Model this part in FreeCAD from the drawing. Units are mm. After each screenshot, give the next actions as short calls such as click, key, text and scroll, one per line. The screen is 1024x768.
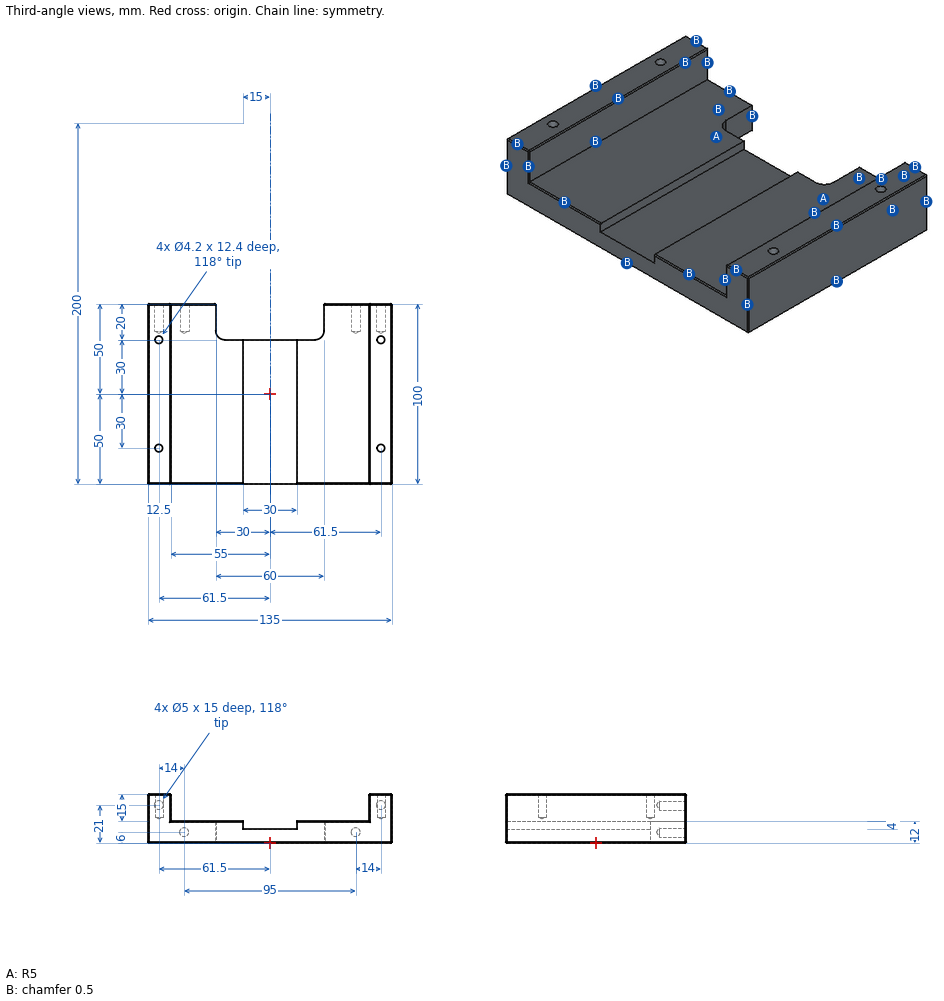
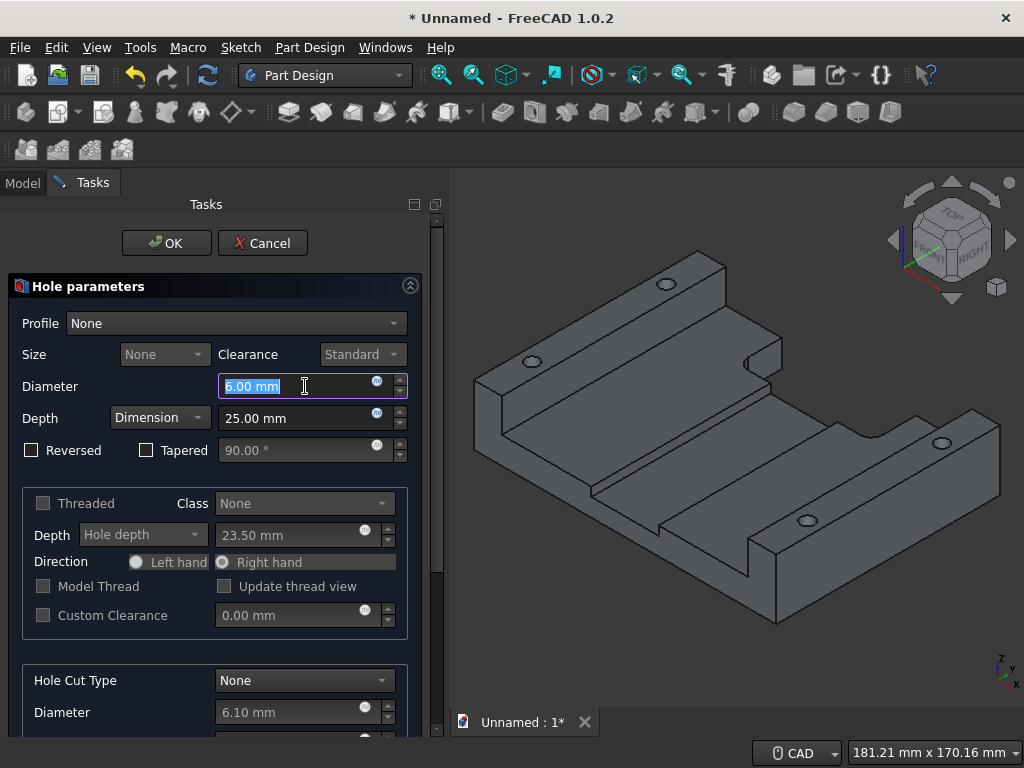
text(4.2)
key(Tab)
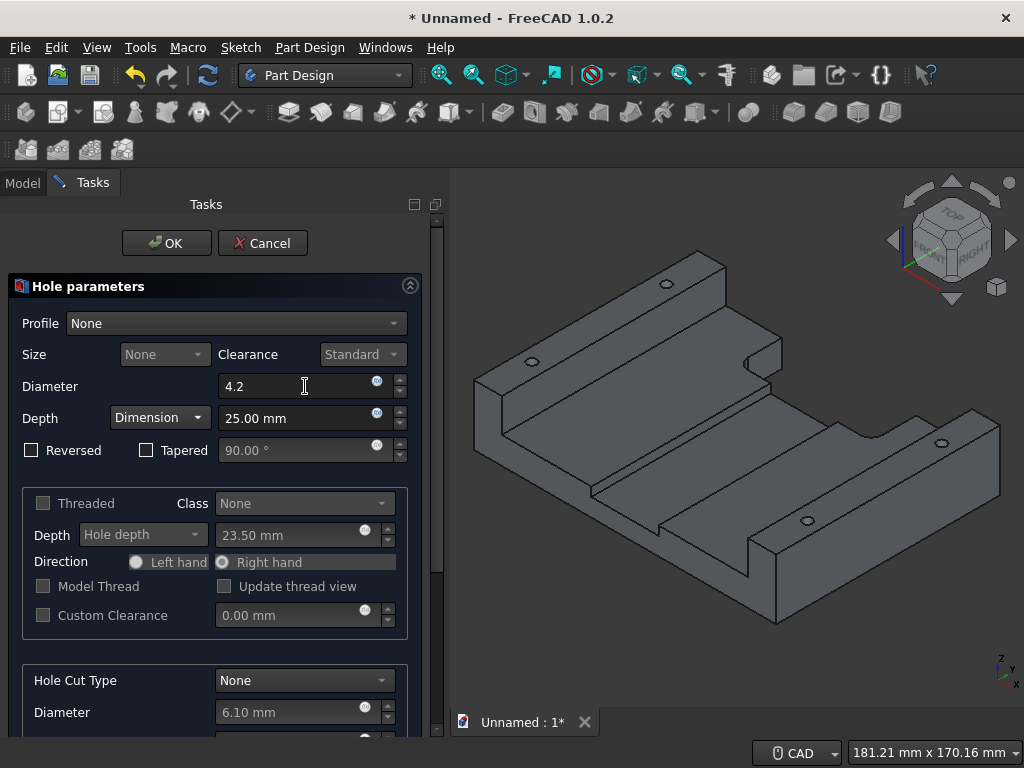
triple_click(305, 418)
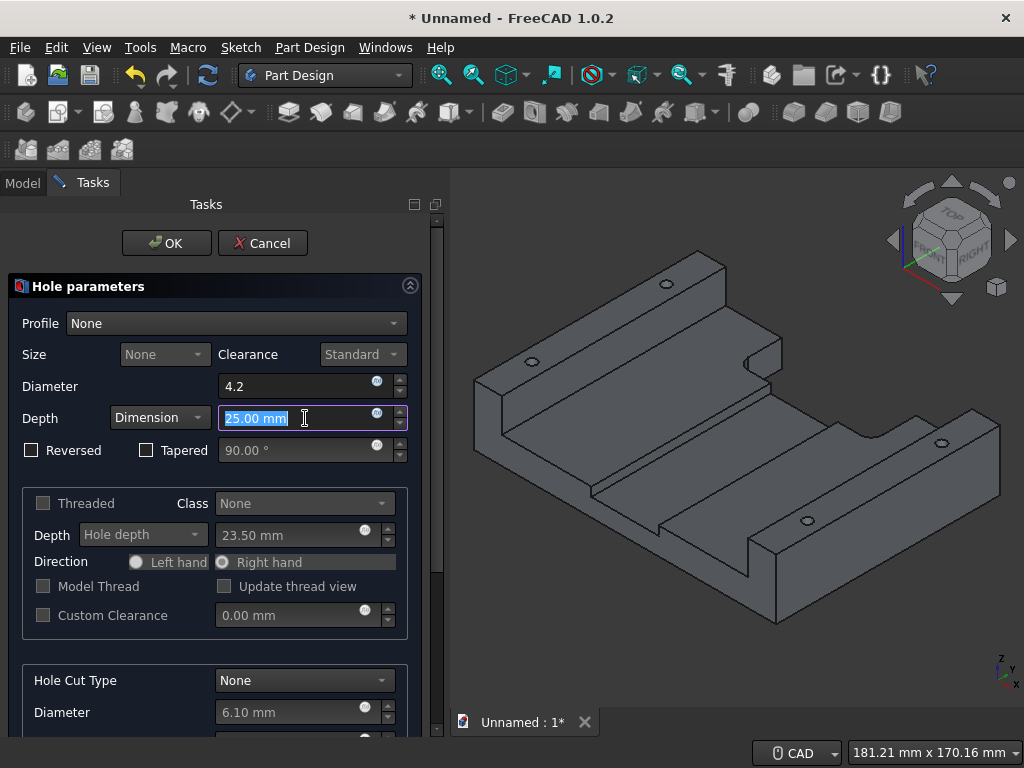
text(12.4)
key(Tab)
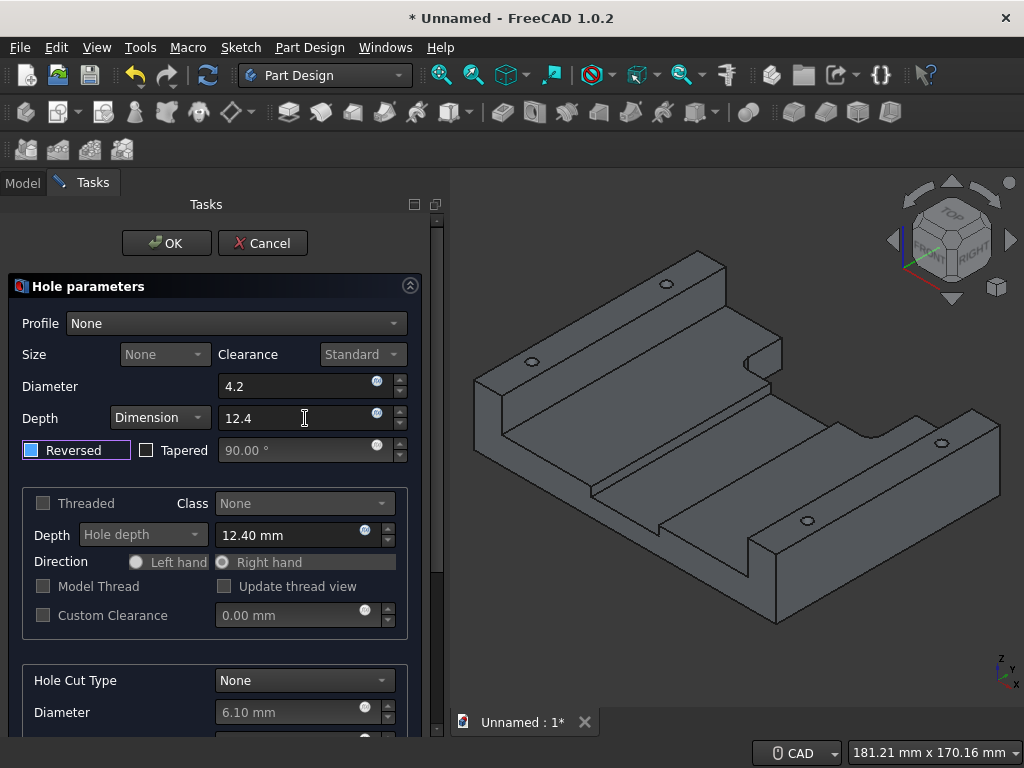
click(167, 243)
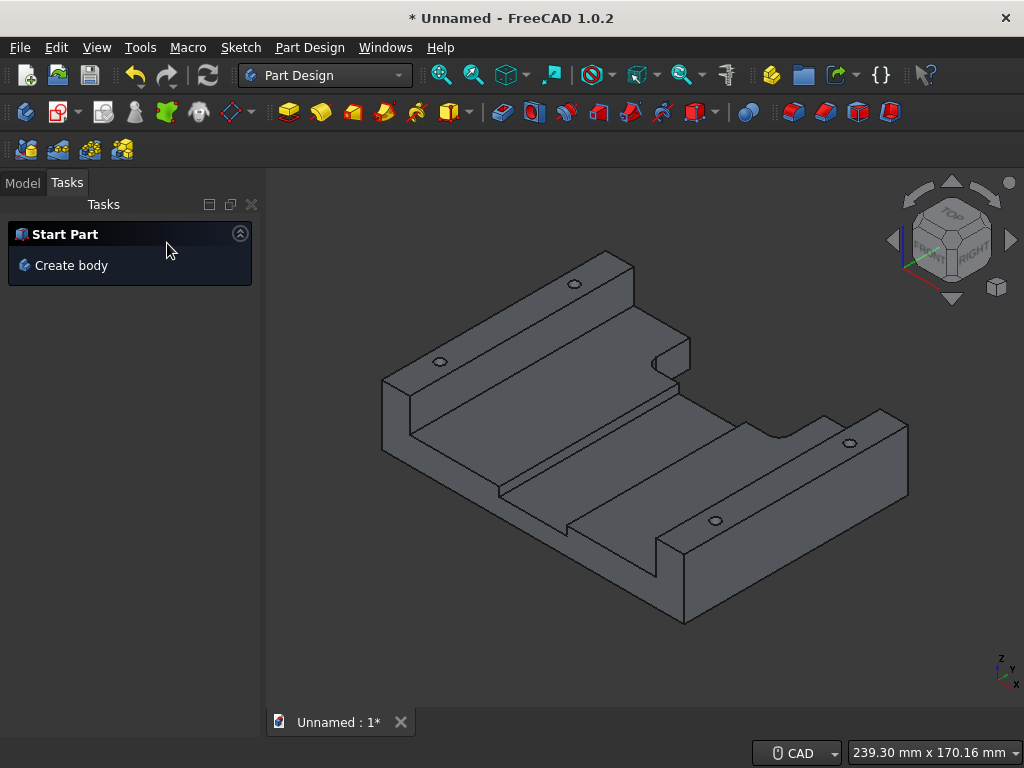
click(860, 487)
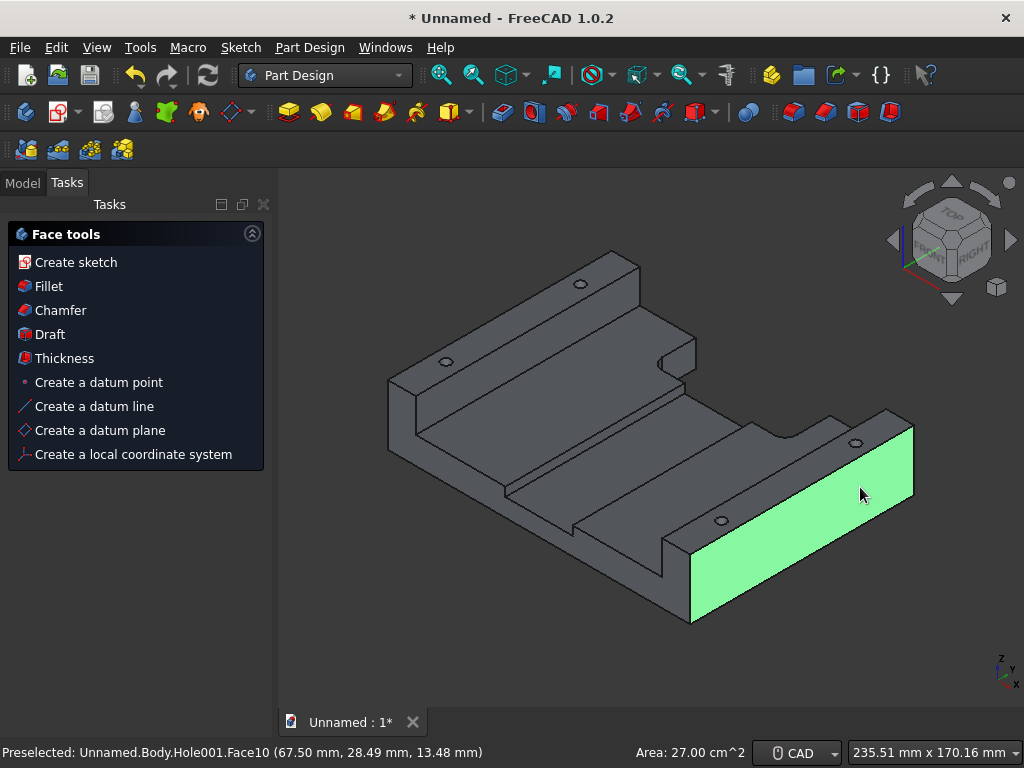
click(461, 460, ctrl)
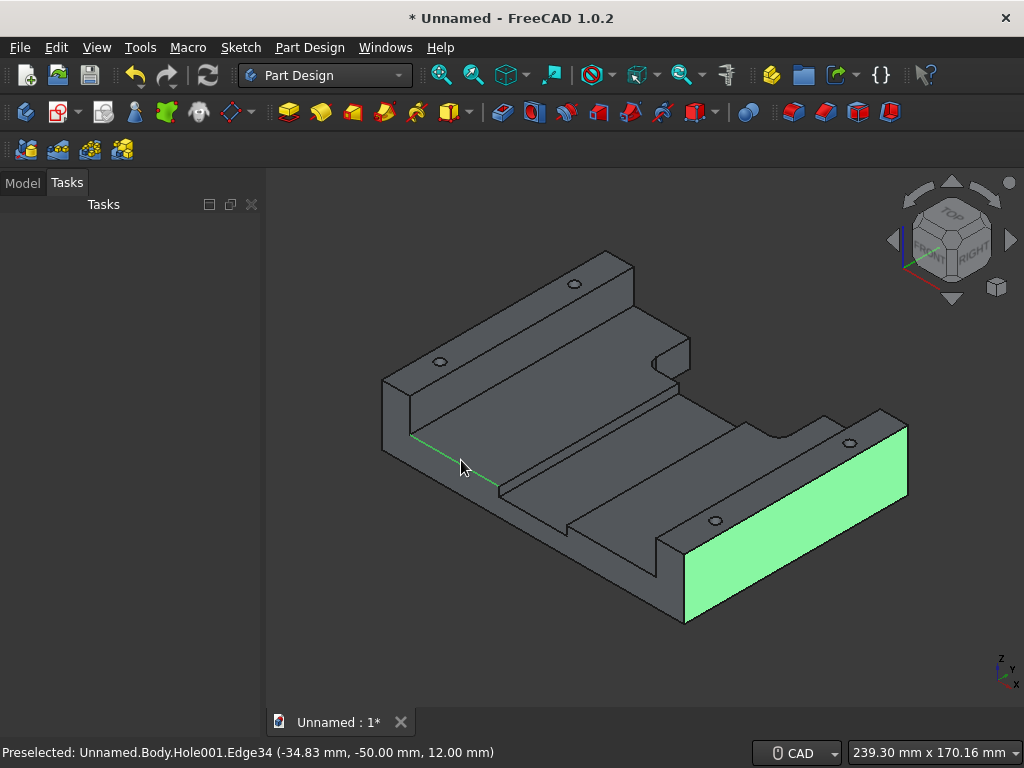
click(410, 415, ctrl)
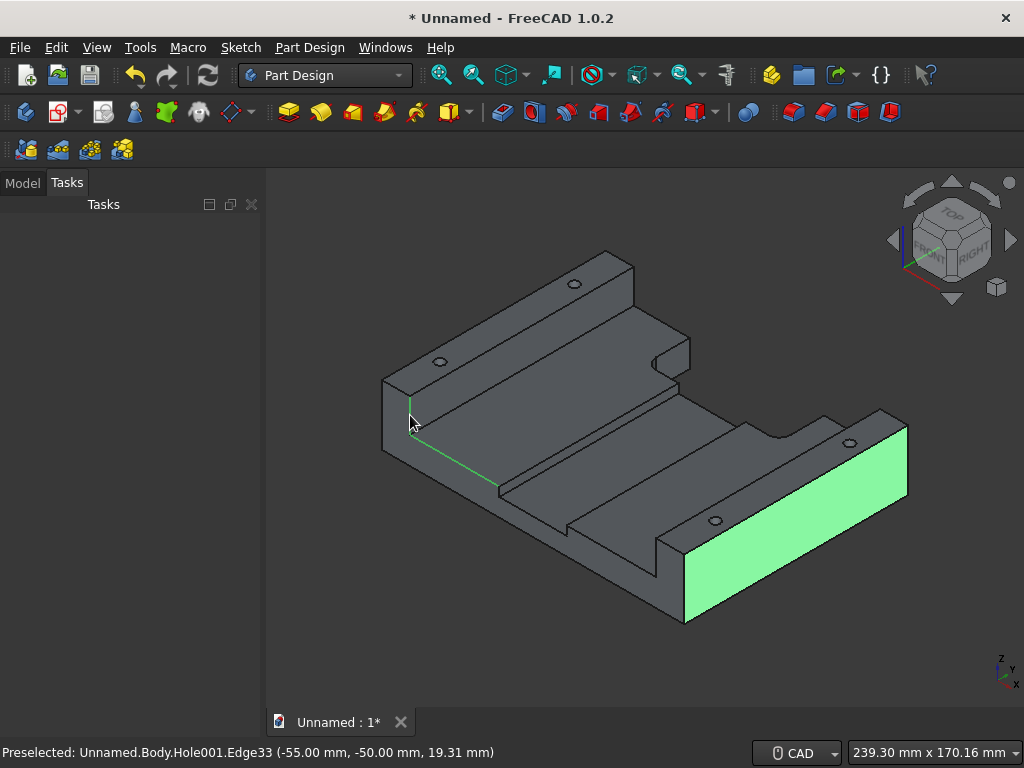
click(396, 387, ctrl)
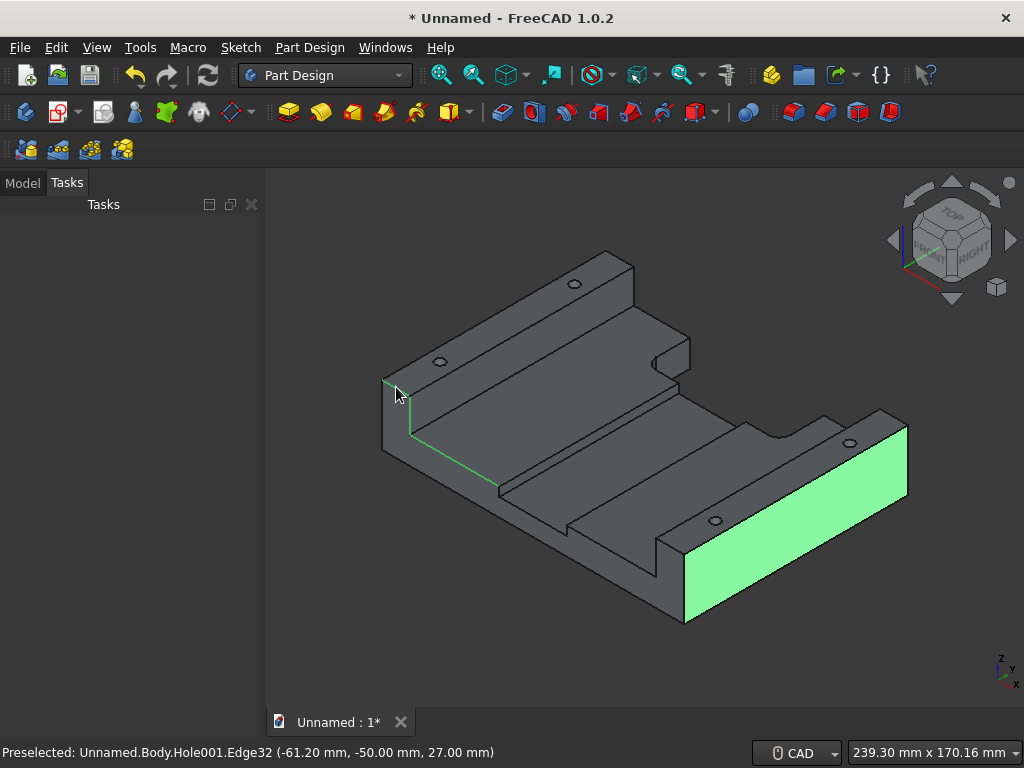
click(522, 330, ctrl)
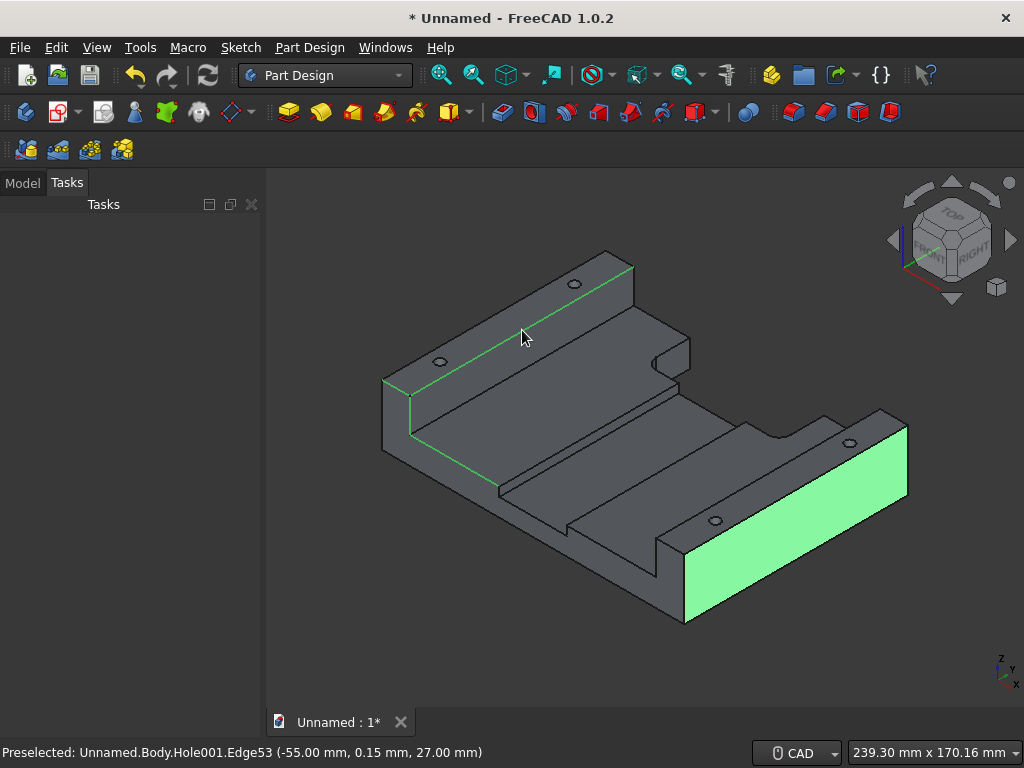
click(670, 545, ctrl)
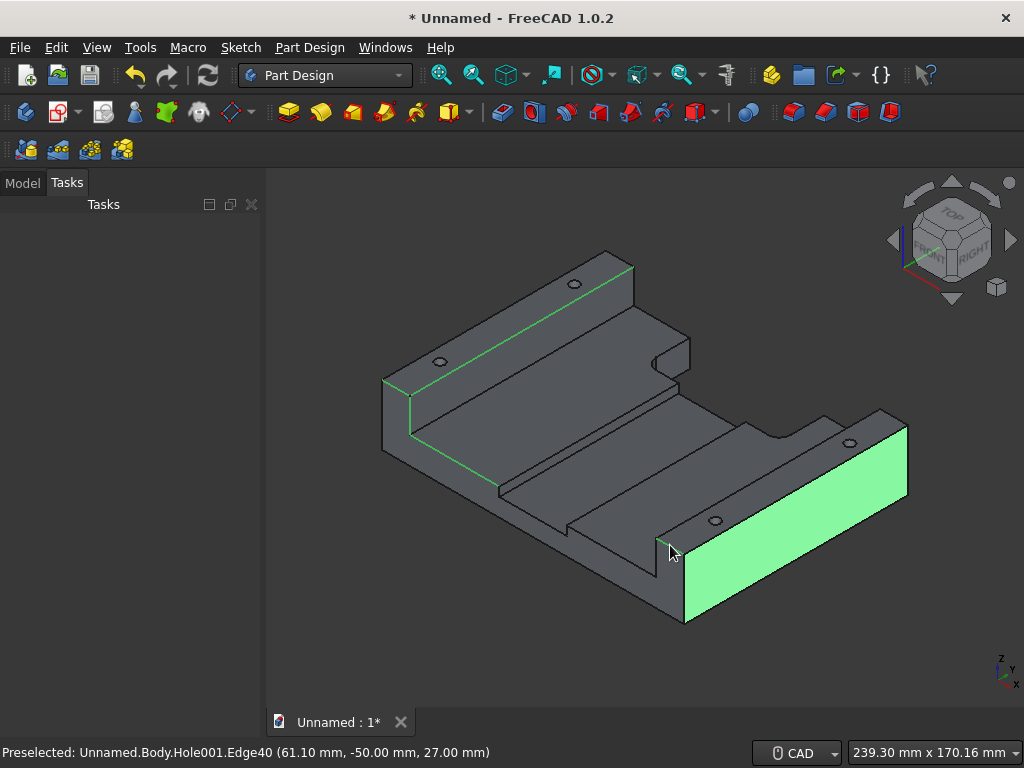
click(611, 550, ctrl)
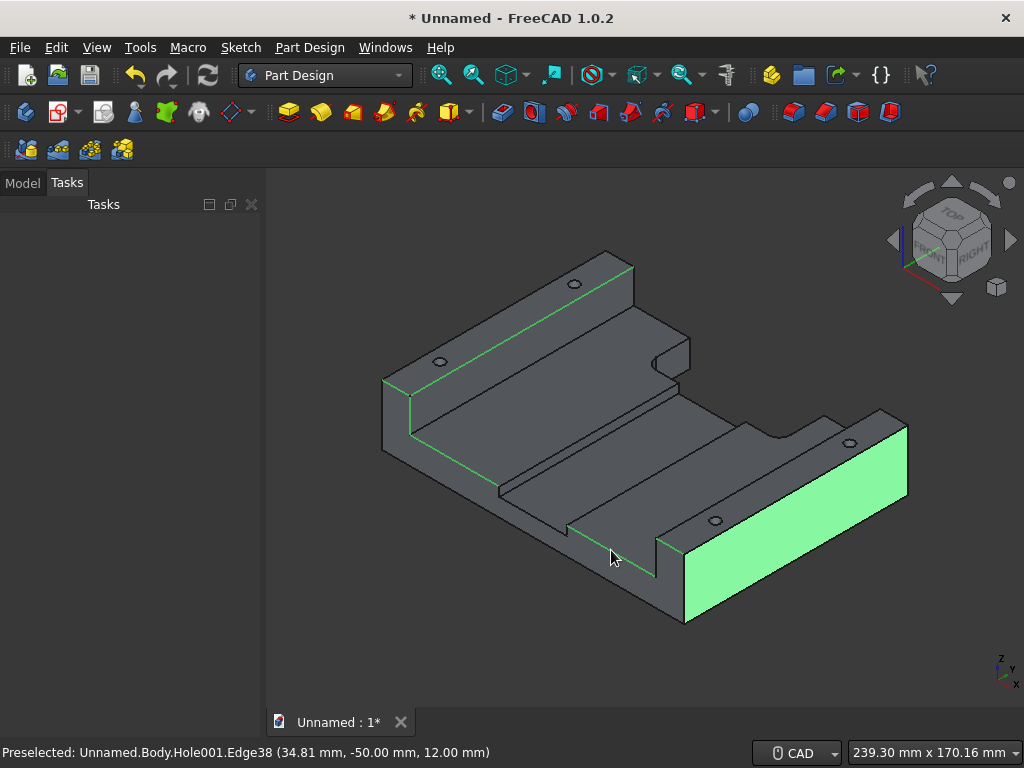
key(2)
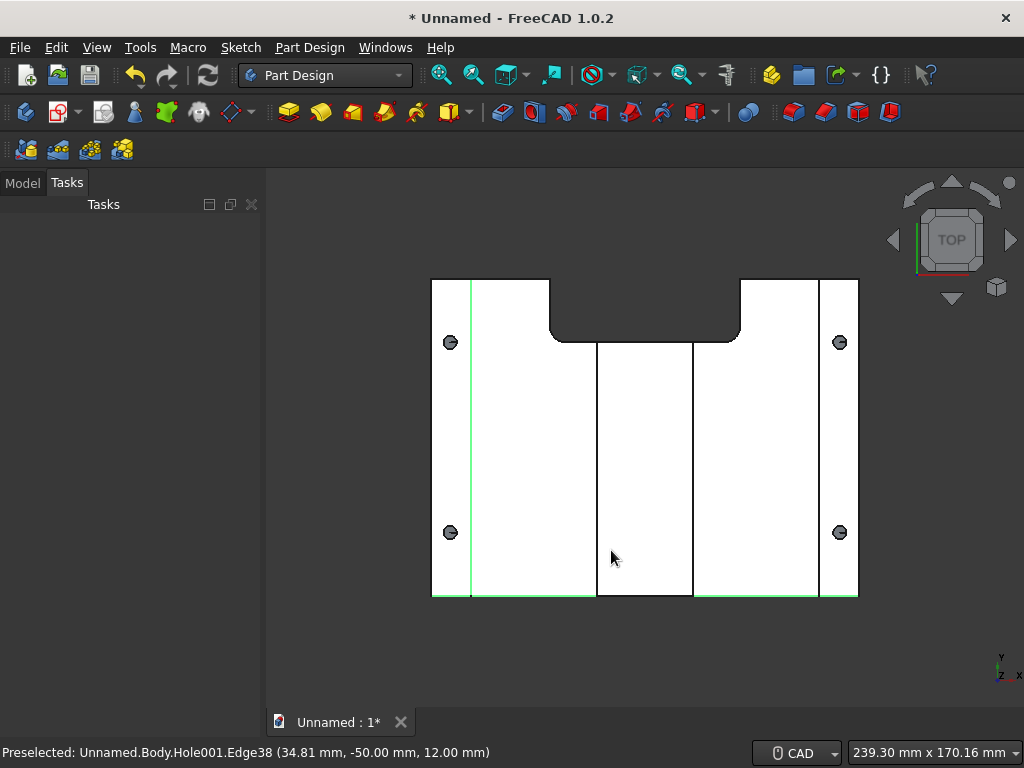
click(451, 278, ctrl)